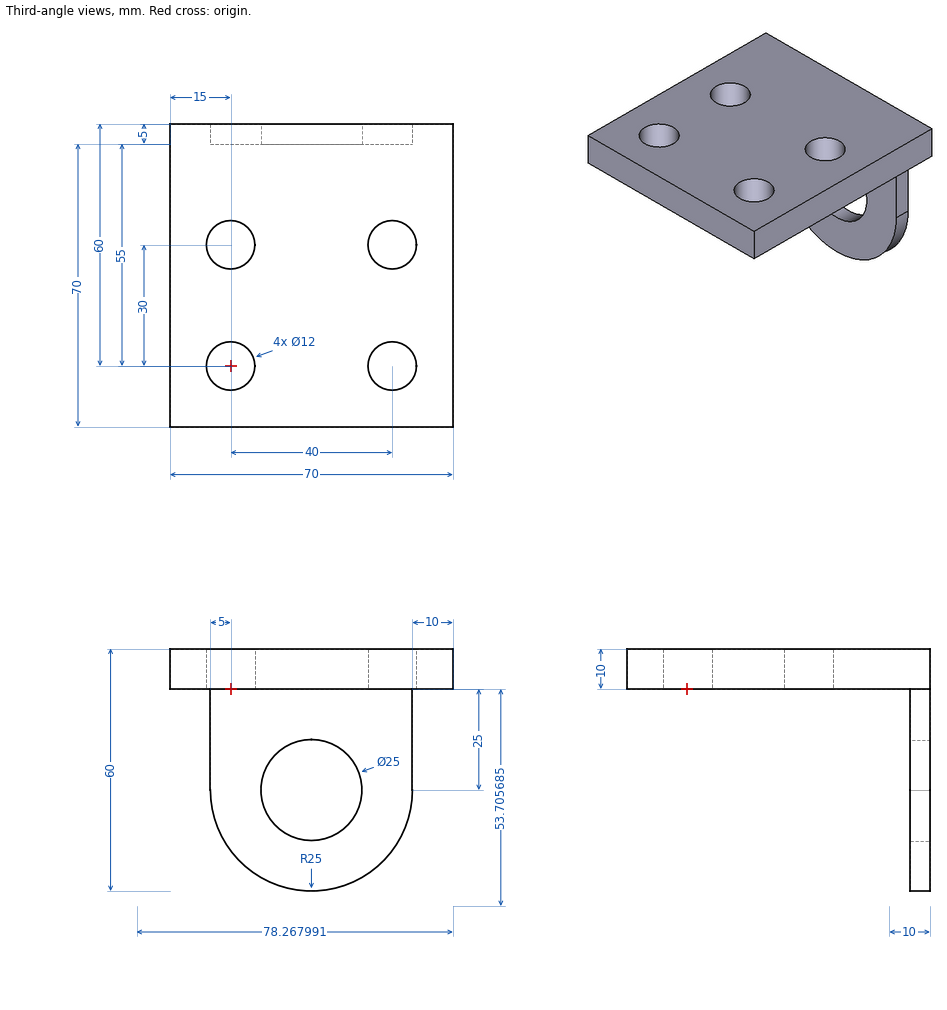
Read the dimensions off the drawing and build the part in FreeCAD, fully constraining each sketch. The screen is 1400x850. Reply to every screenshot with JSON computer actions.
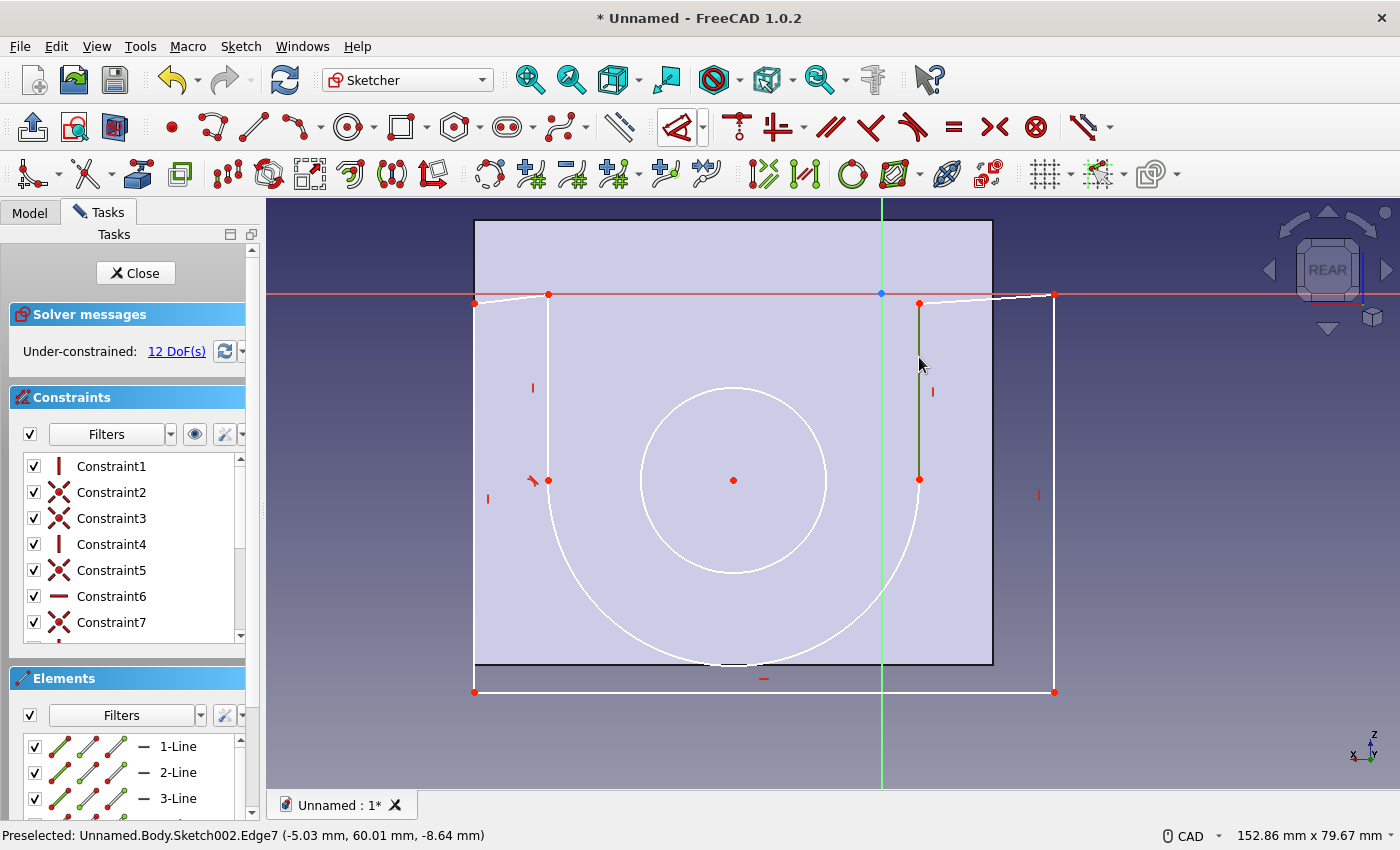
{"action": "left_click", "coordinate": [625, 631]}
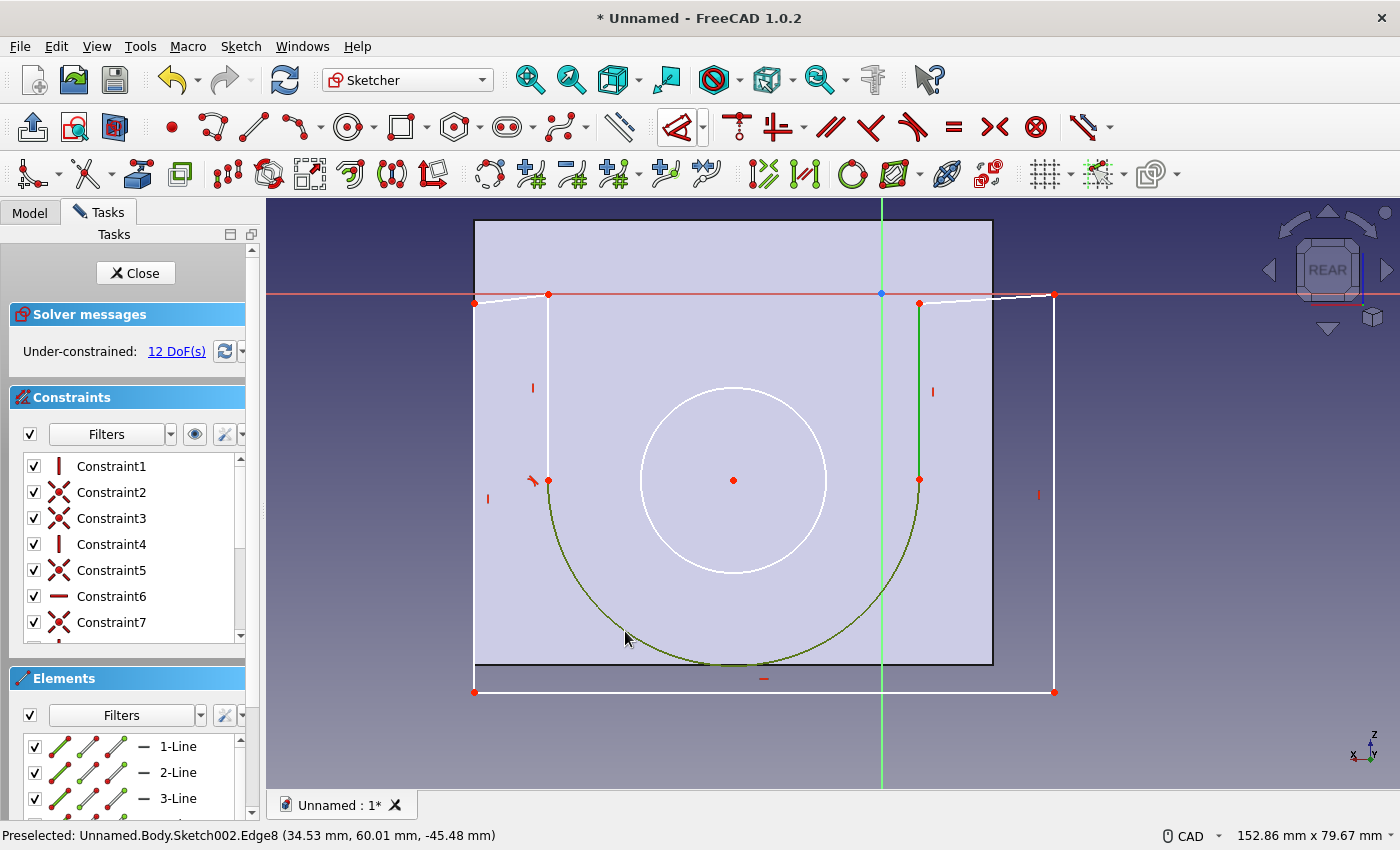
{"action": "left_click", "coordinate": [913, 128]}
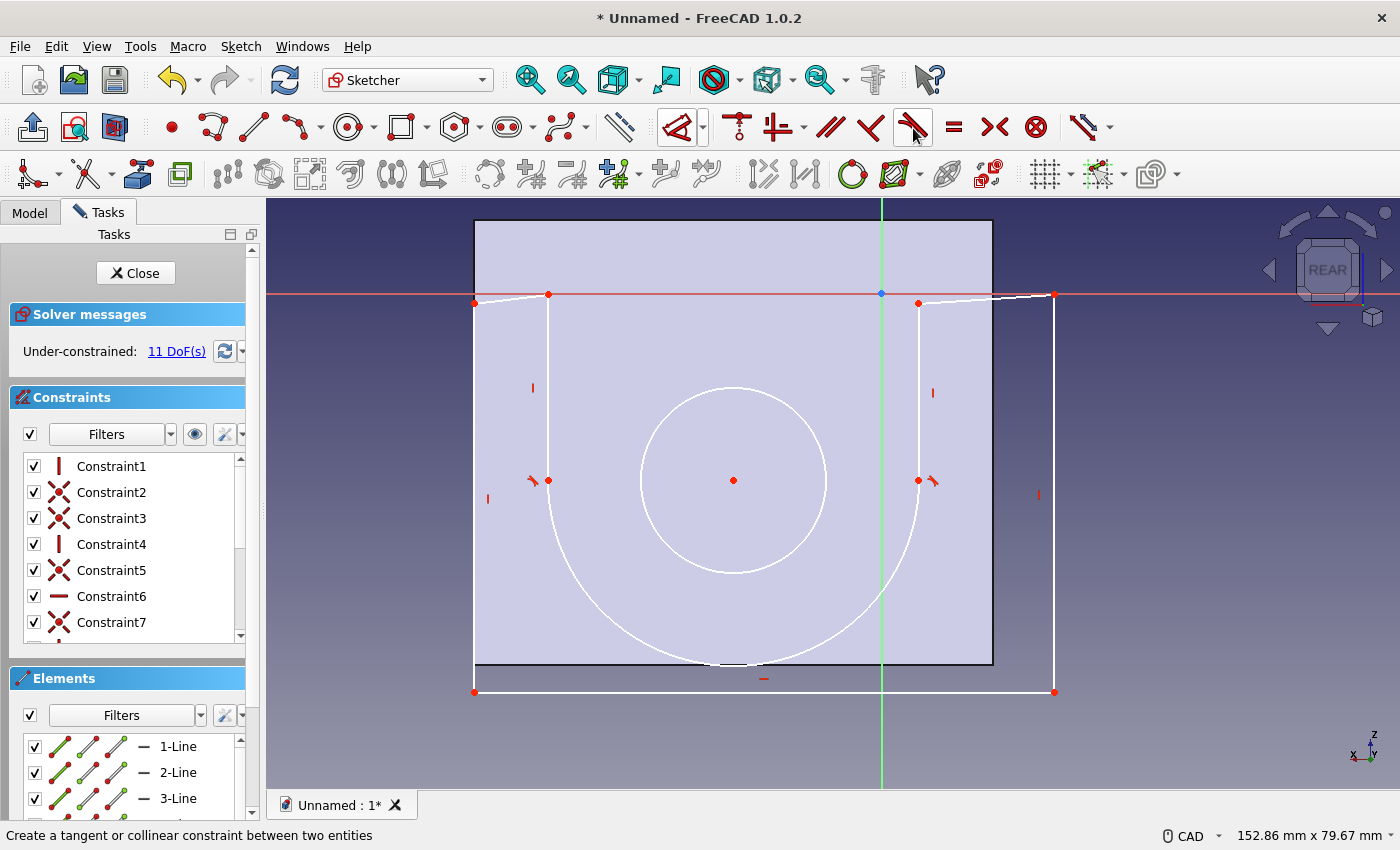
{"action": "left_click", "coordinate": [526, 298]}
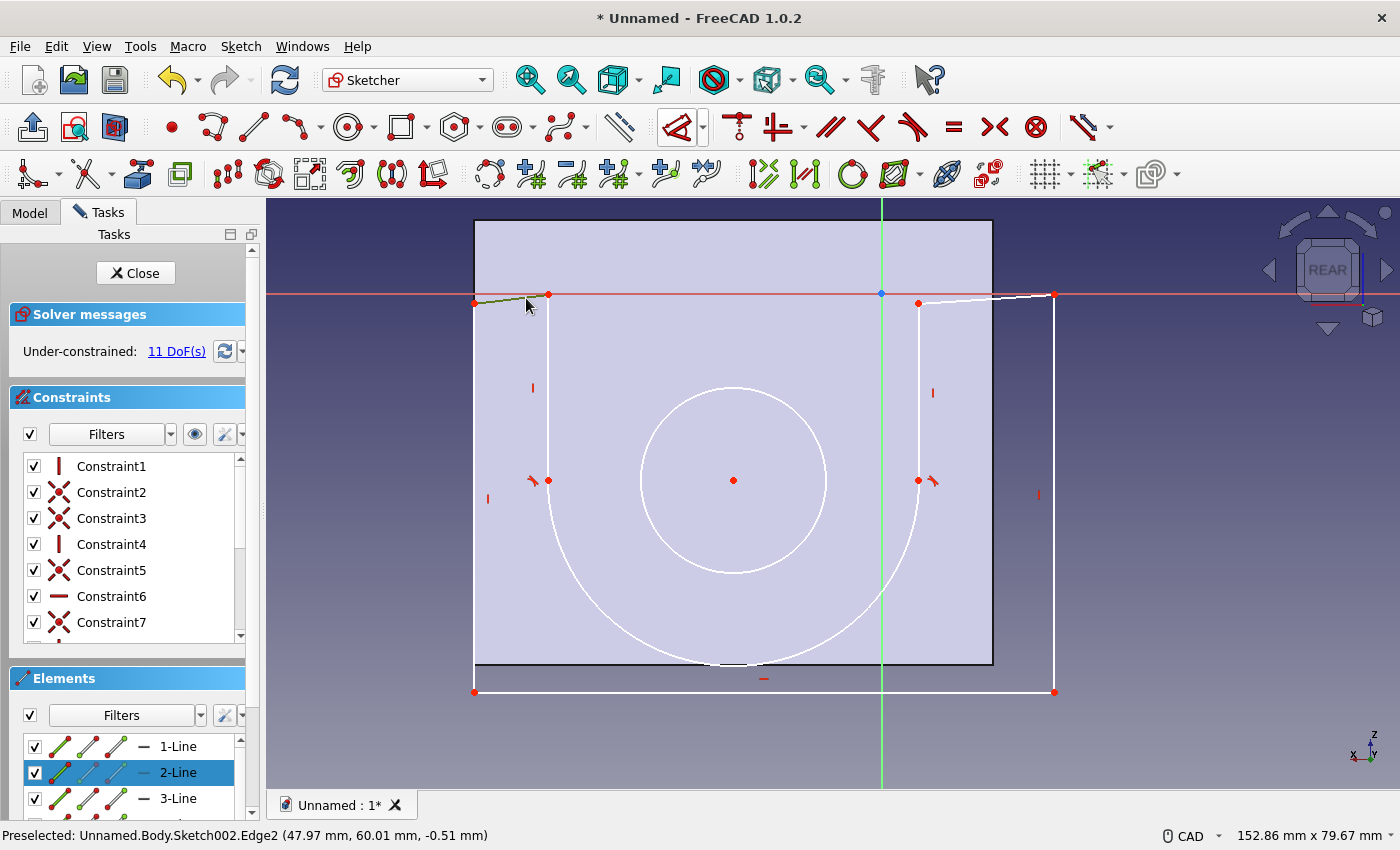
{"action": "left_click", "coordinate": [804, 128]}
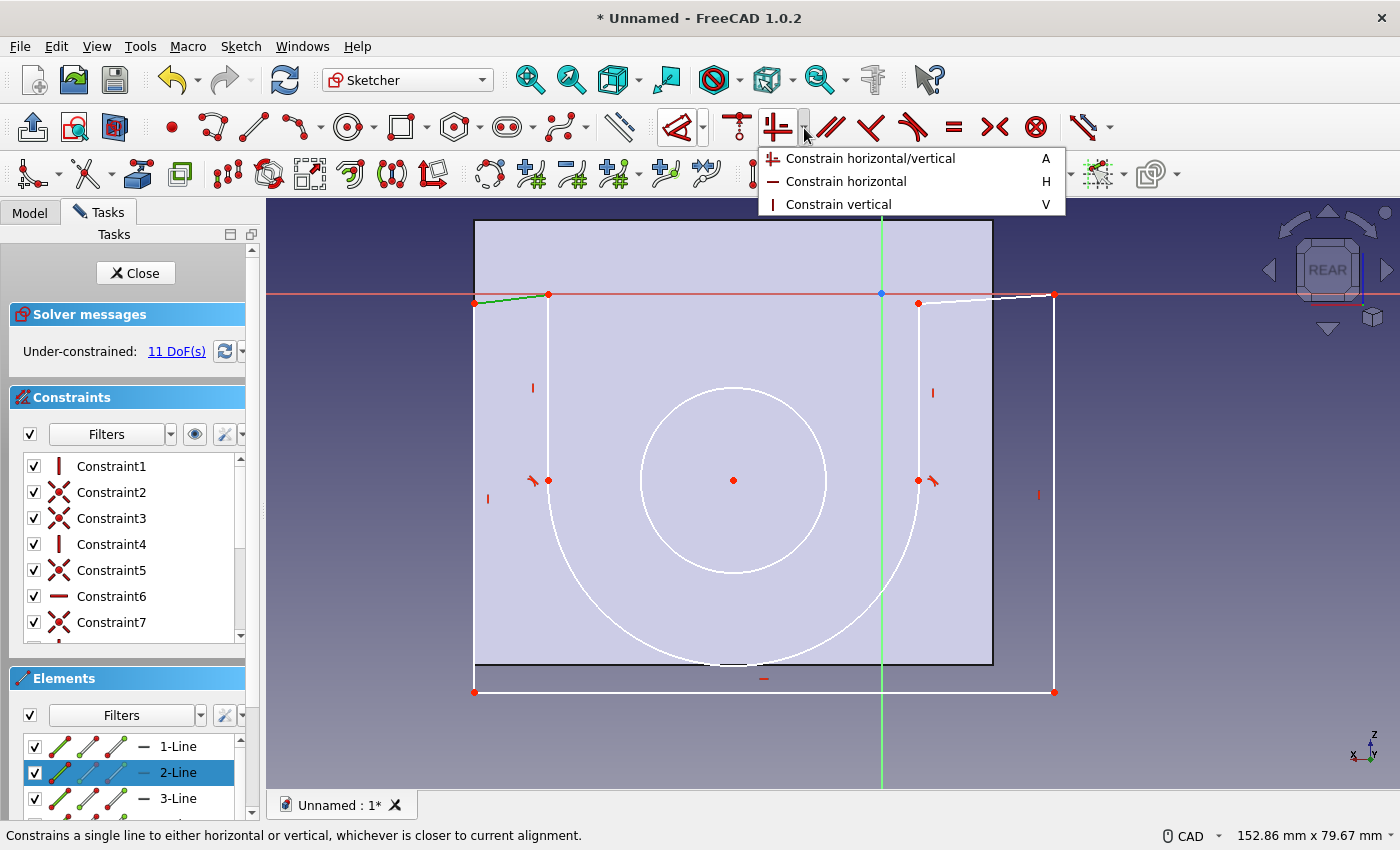
{"action": "left_click", "coordinate": [912, 182]}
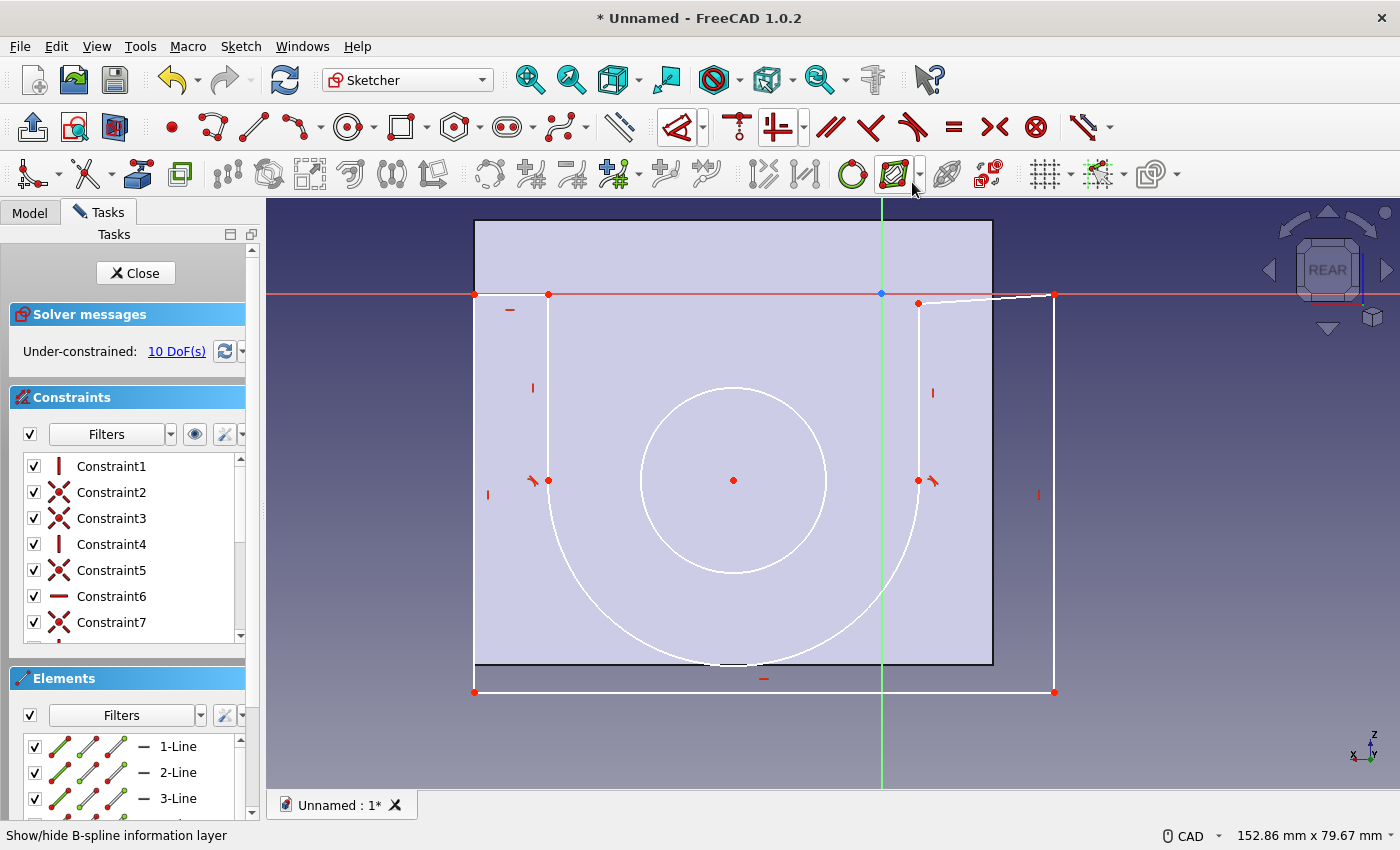
{"action": "left_click", "coordinate": [1013, 298]}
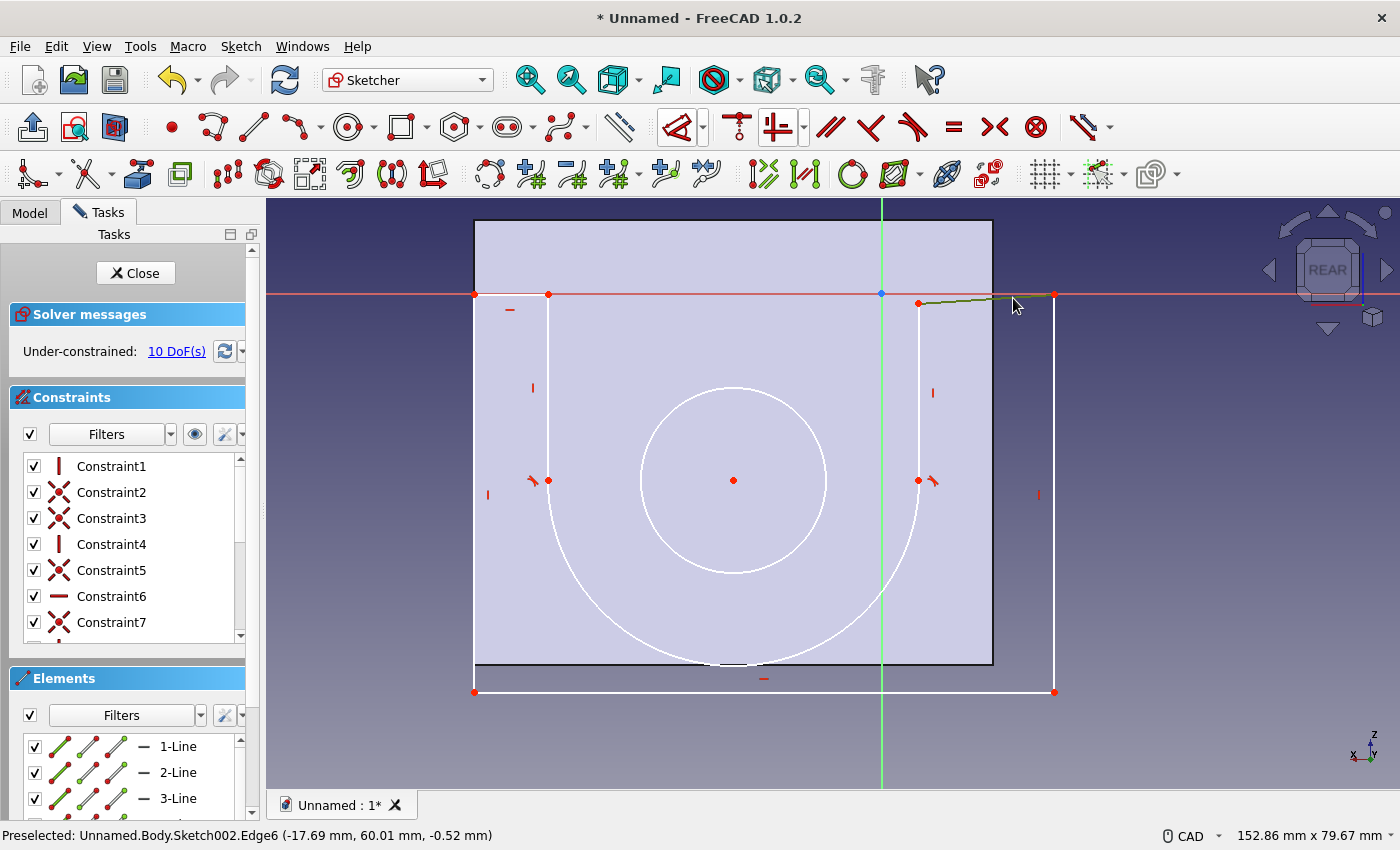
{"action": "left_click", "coordinate": [804, 128]}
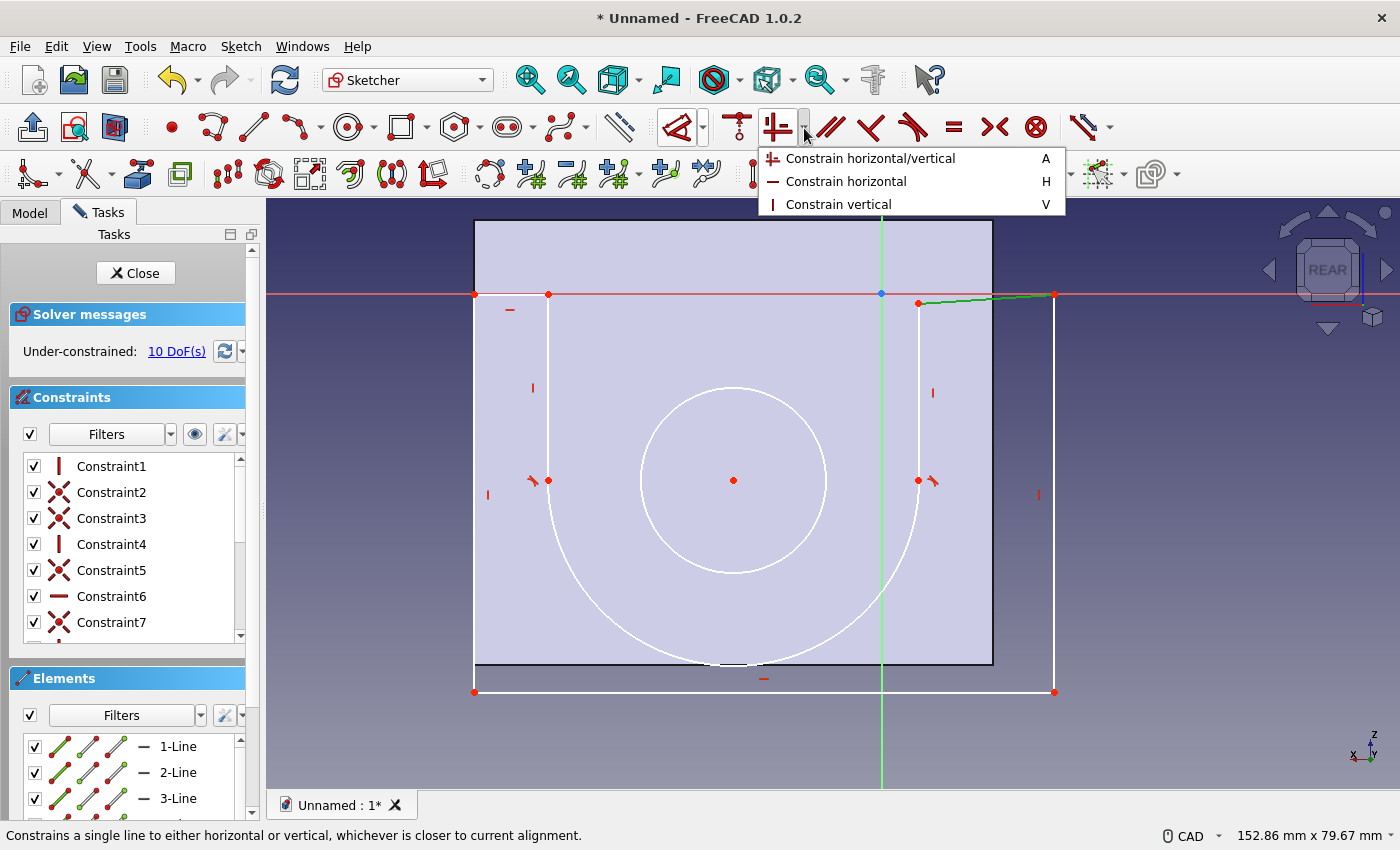
{"action": "left_click", "coordinate": [912, 182]}